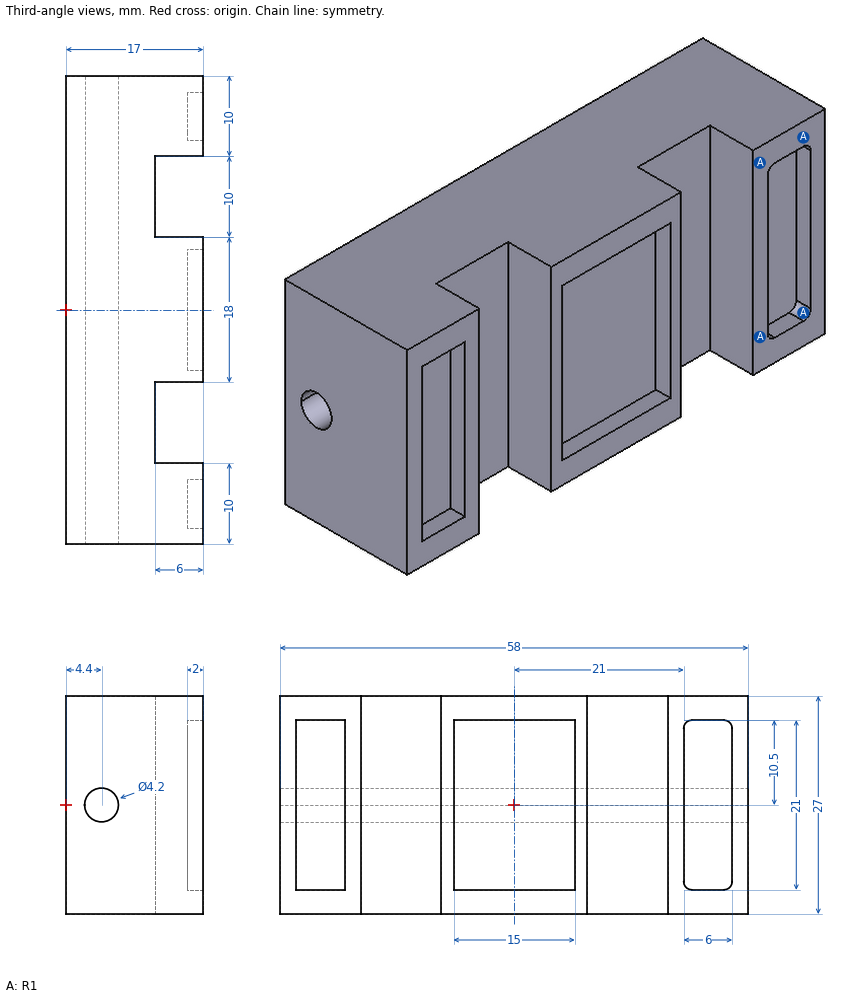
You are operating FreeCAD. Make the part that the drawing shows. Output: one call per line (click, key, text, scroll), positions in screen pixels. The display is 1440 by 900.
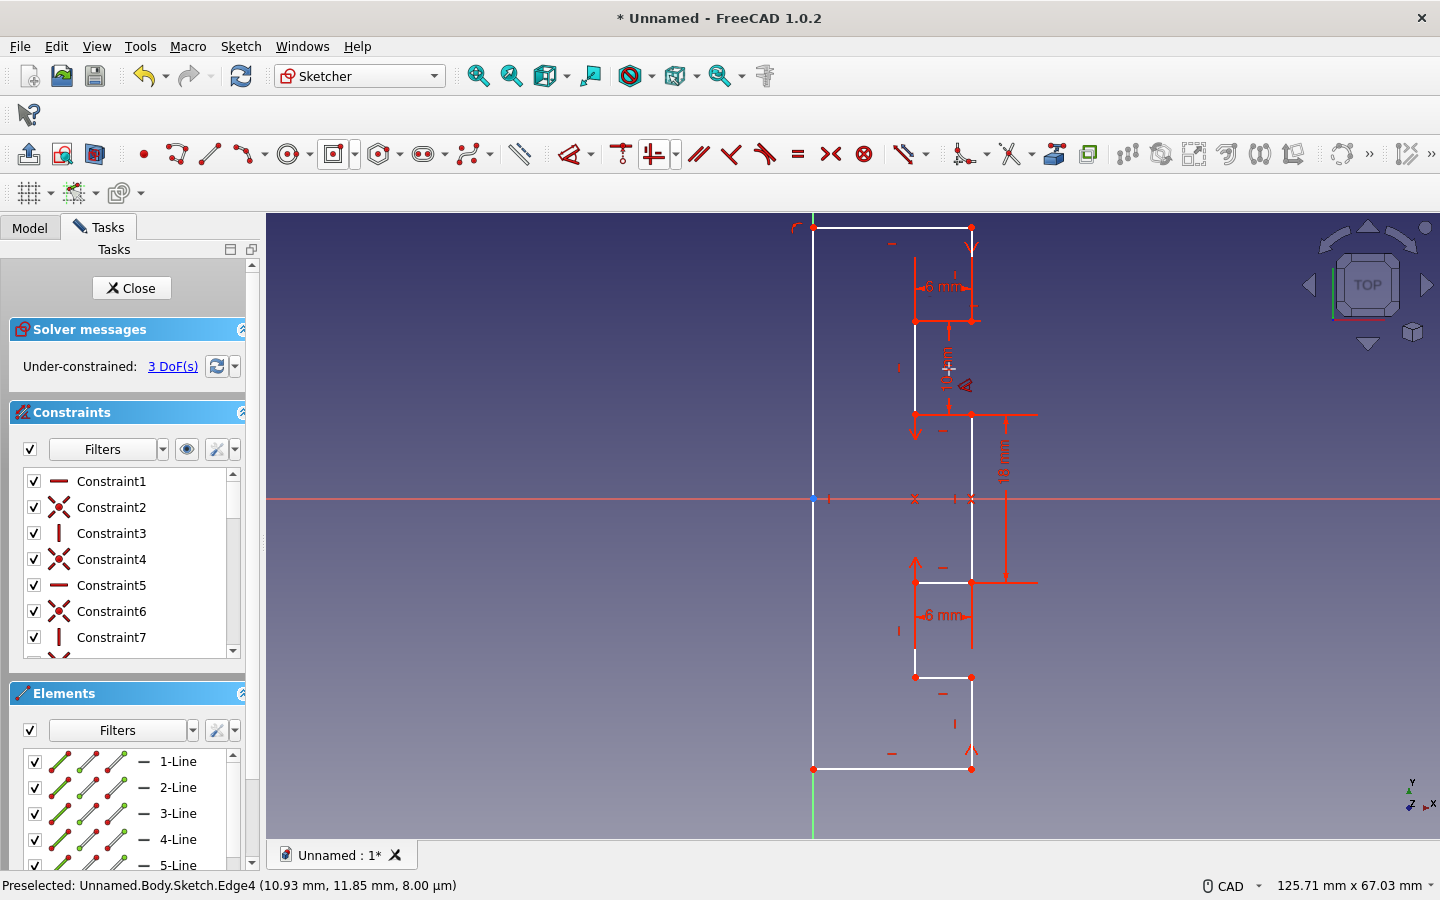
click(972, 293)
click(1006, 263)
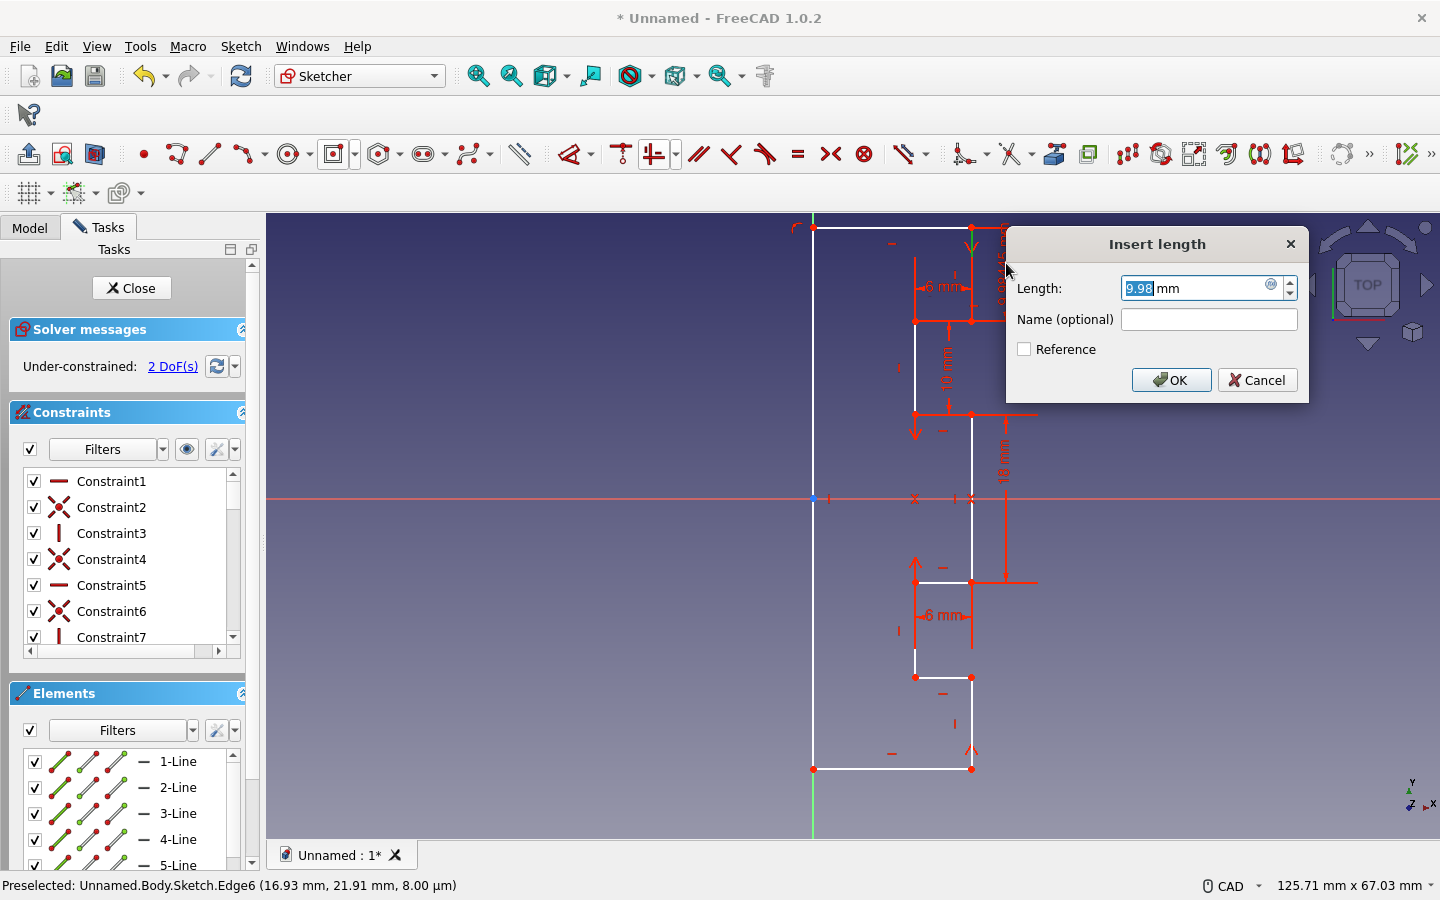
text(10)
key(Return)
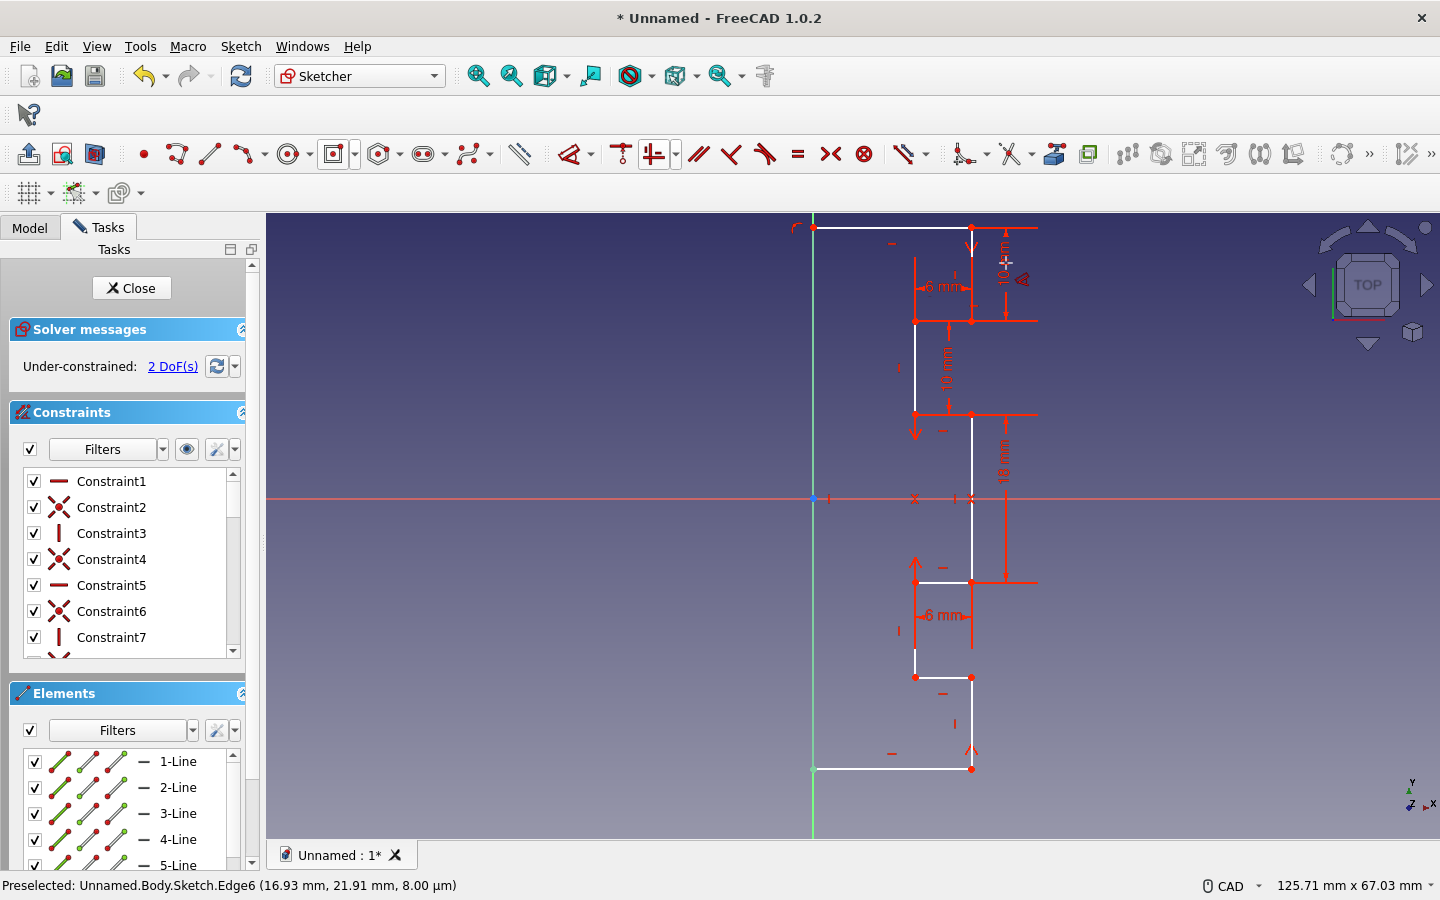
scroll(296, 649, down, 1)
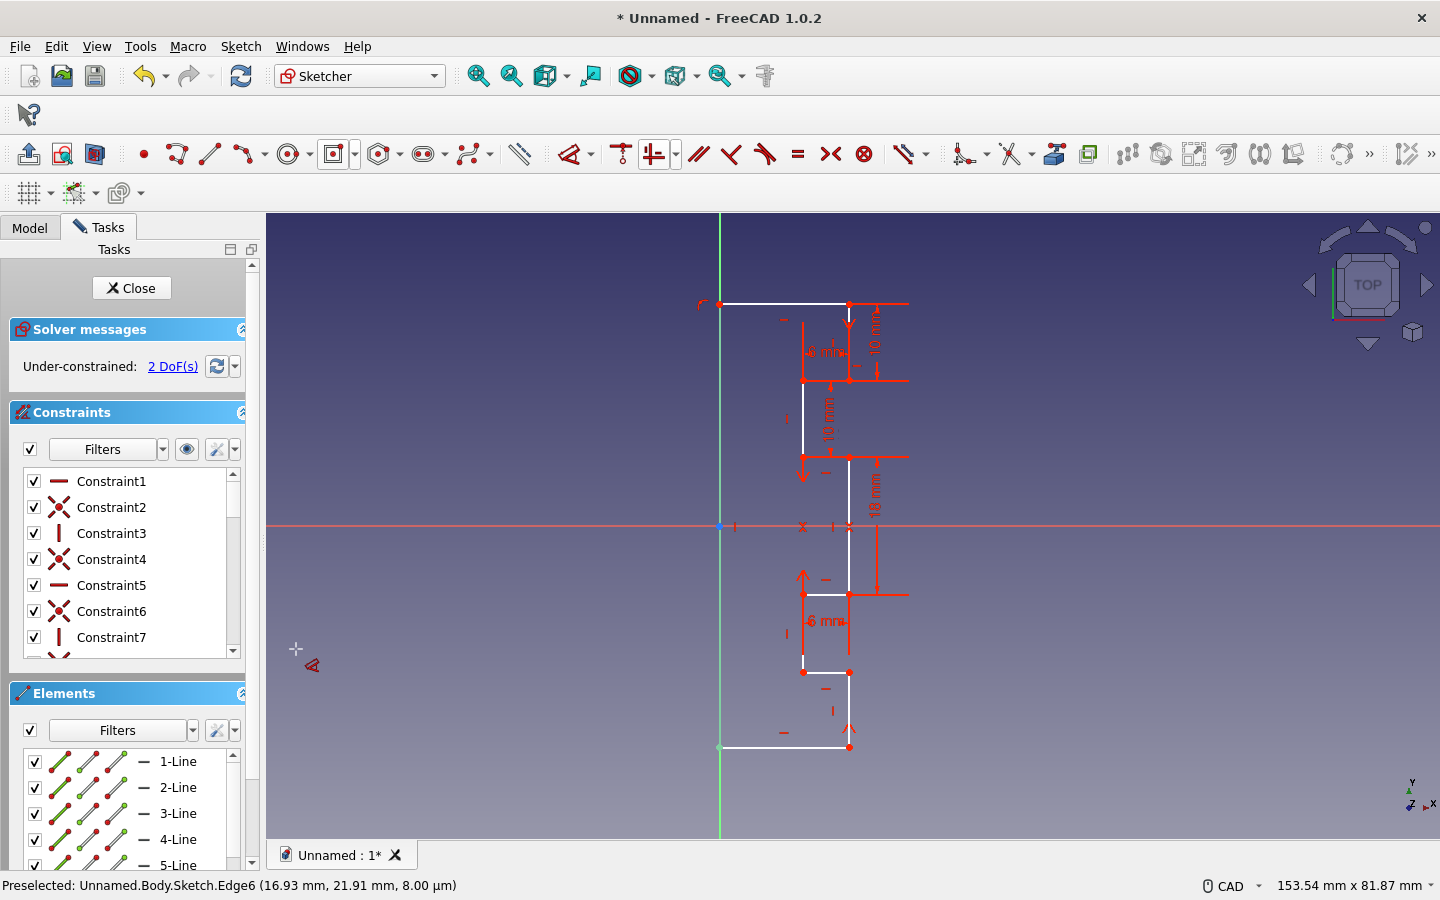
click(810, 304)
click(784, 270)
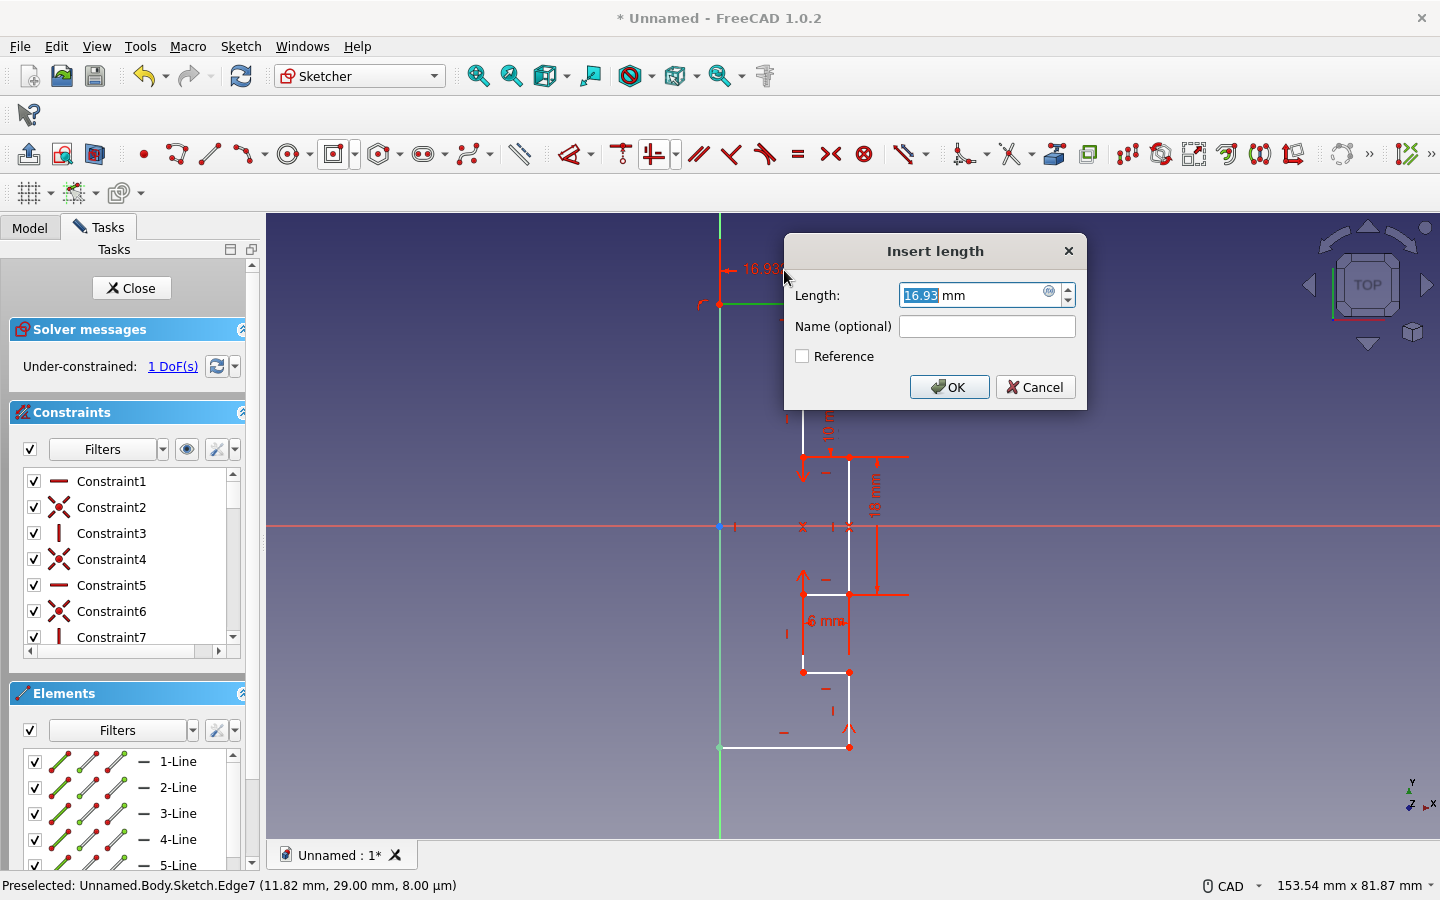
text(17)
key(Return)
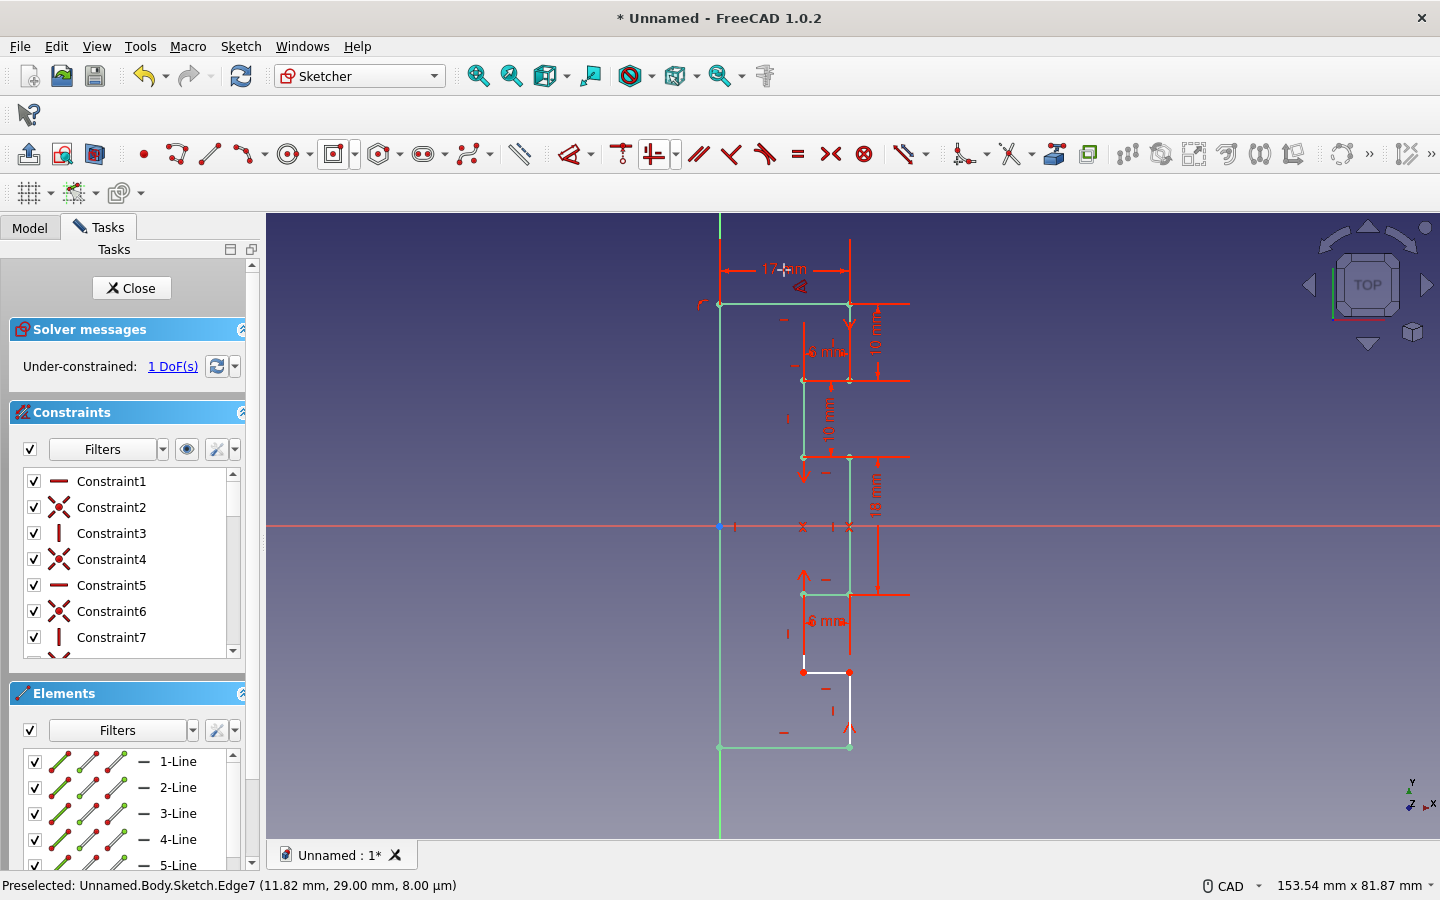
click(850, 725)
click(884, 710)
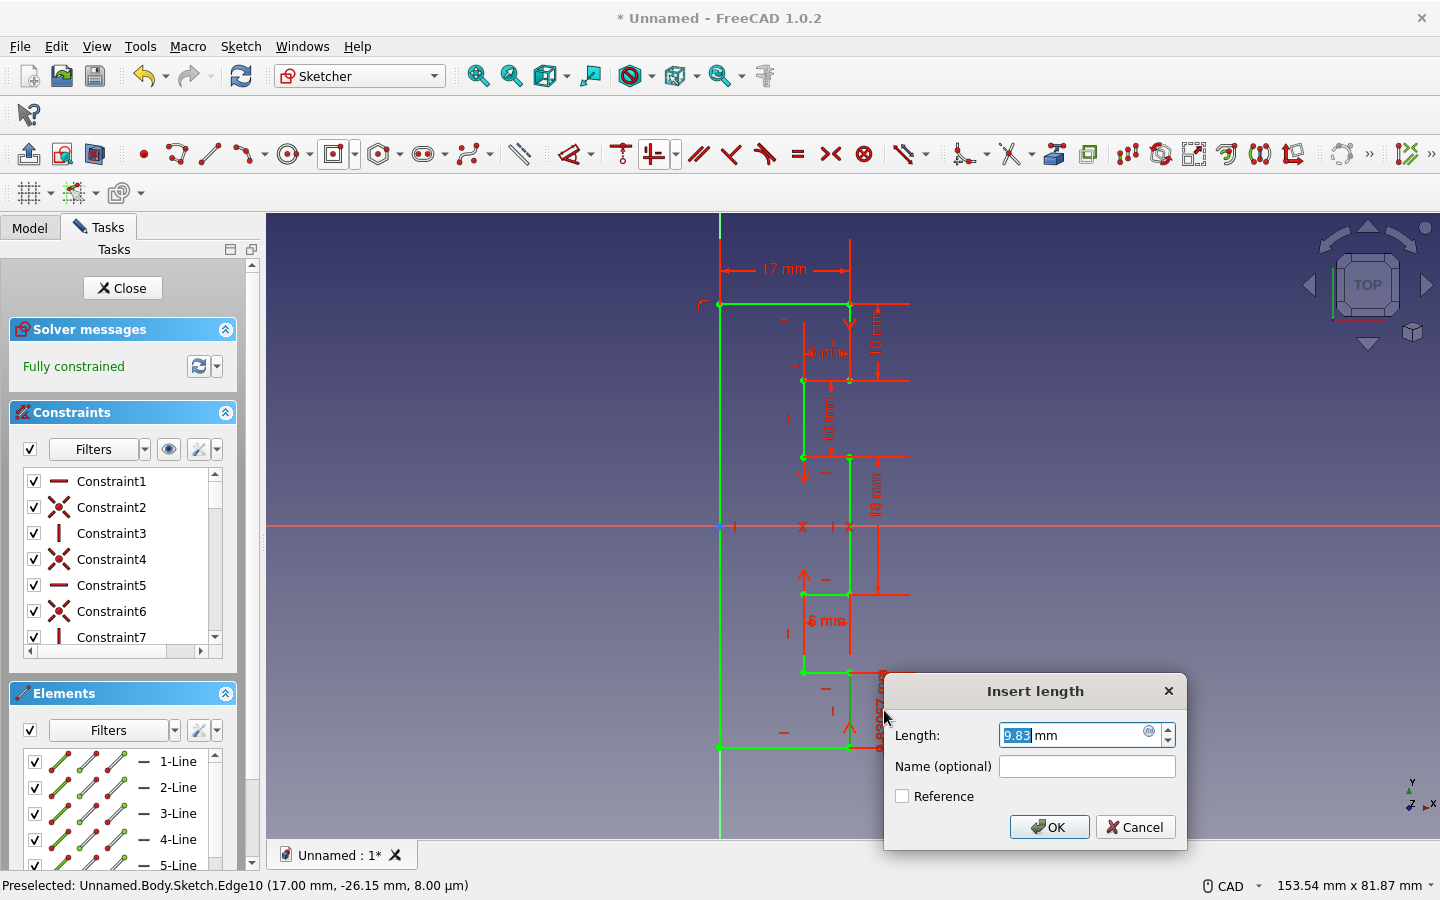
text(10)
key(Return)
key(Escape)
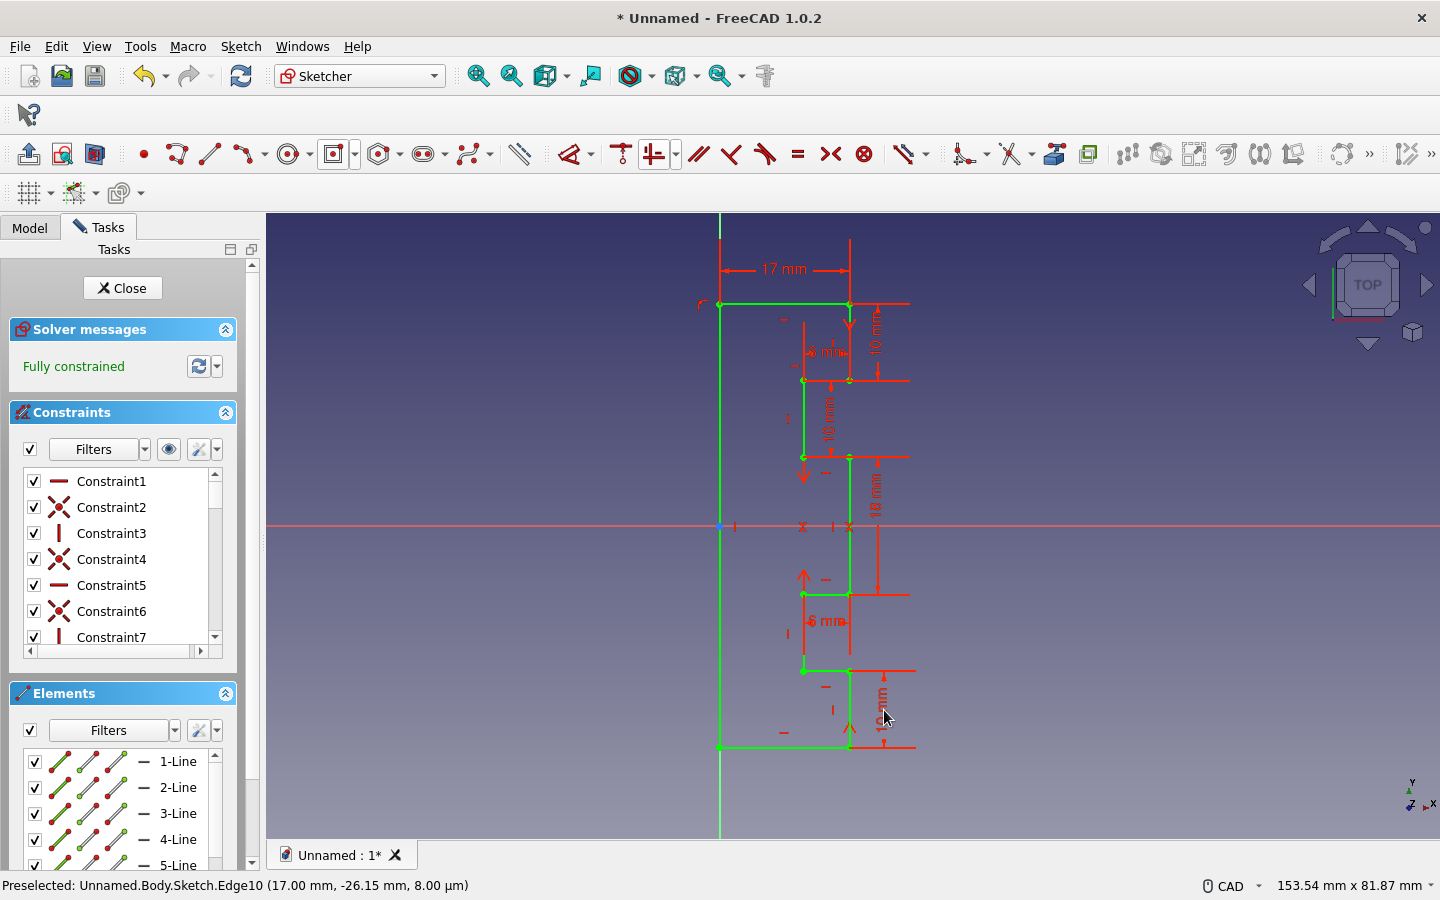
click(123, 288)